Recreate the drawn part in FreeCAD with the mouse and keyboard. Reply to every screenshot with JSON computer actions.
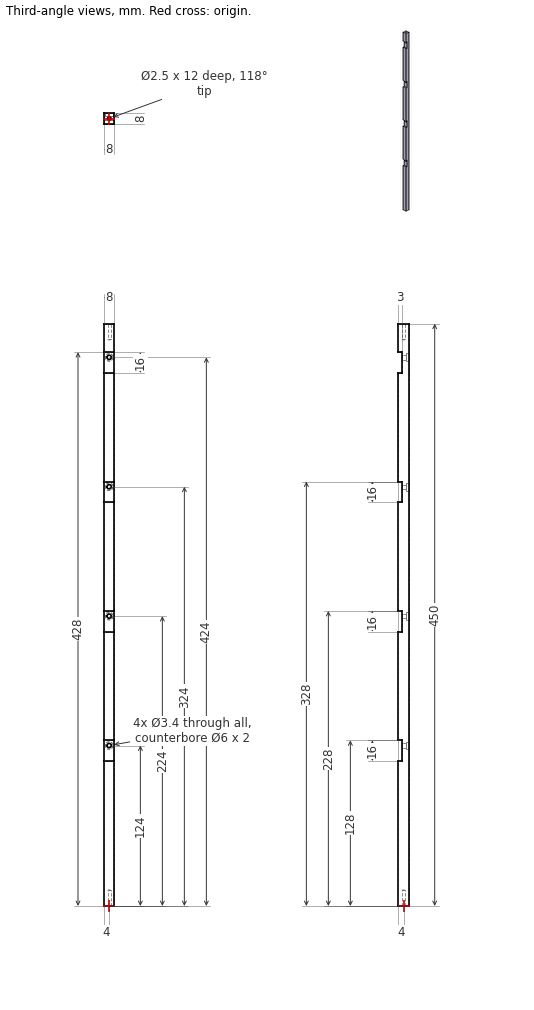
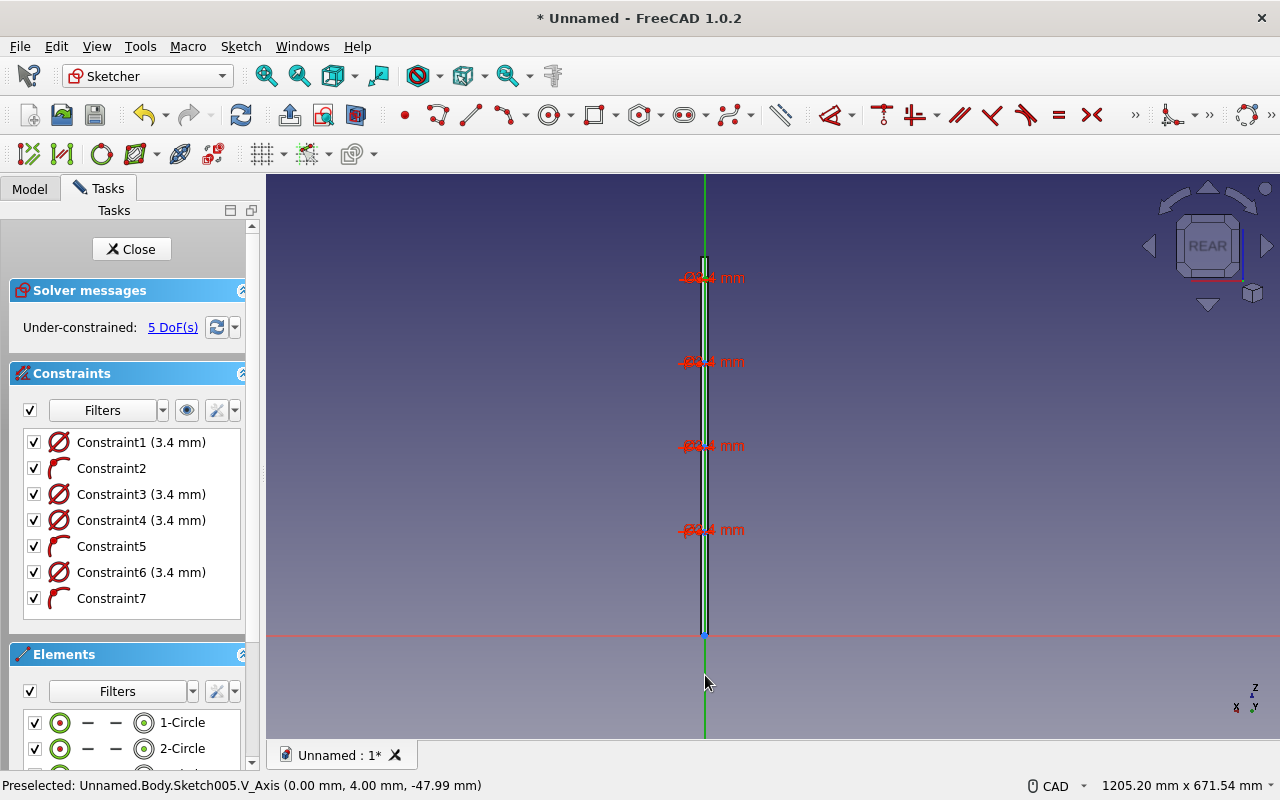
{"action": "key", "text": "c"}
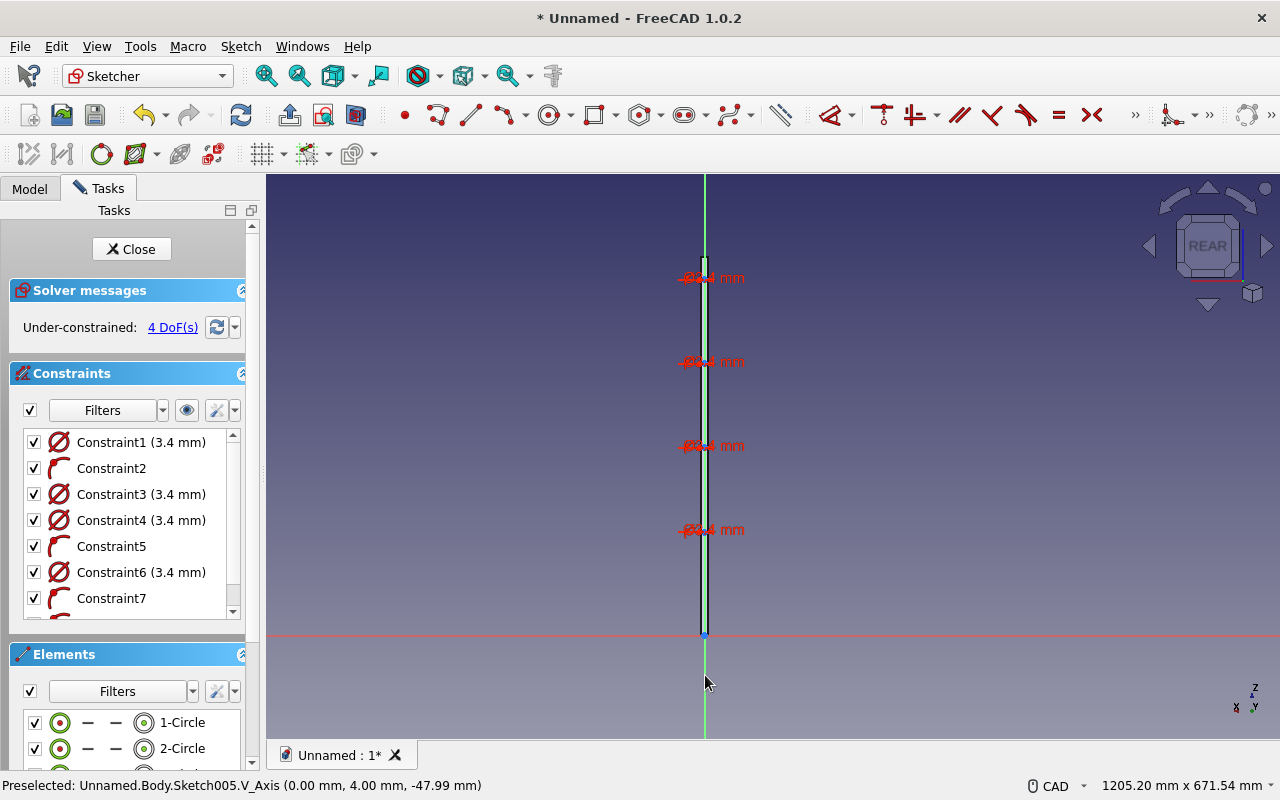
{"action": "key", "text": "d"}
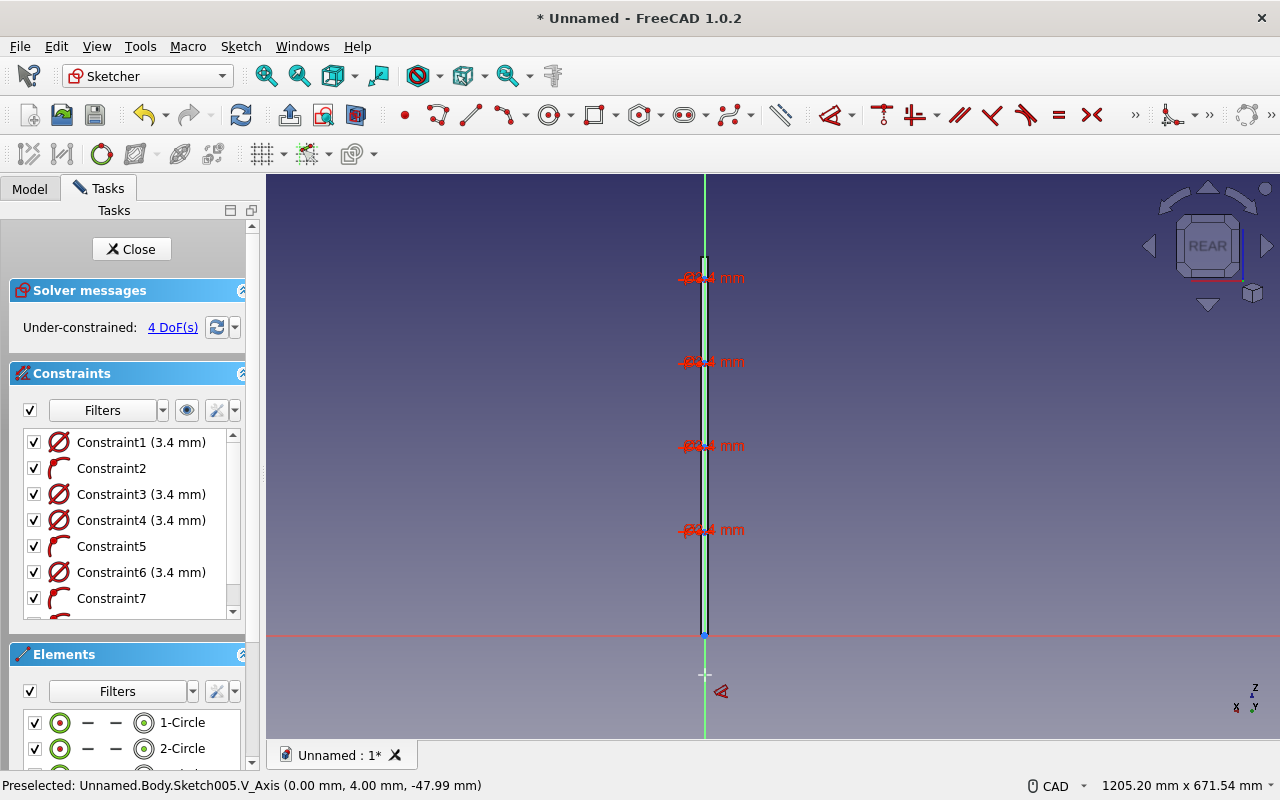
{"action": "left_click", "coordinate": [705, 532]}
{"action": "left_click", "coordinate": [739, 584]}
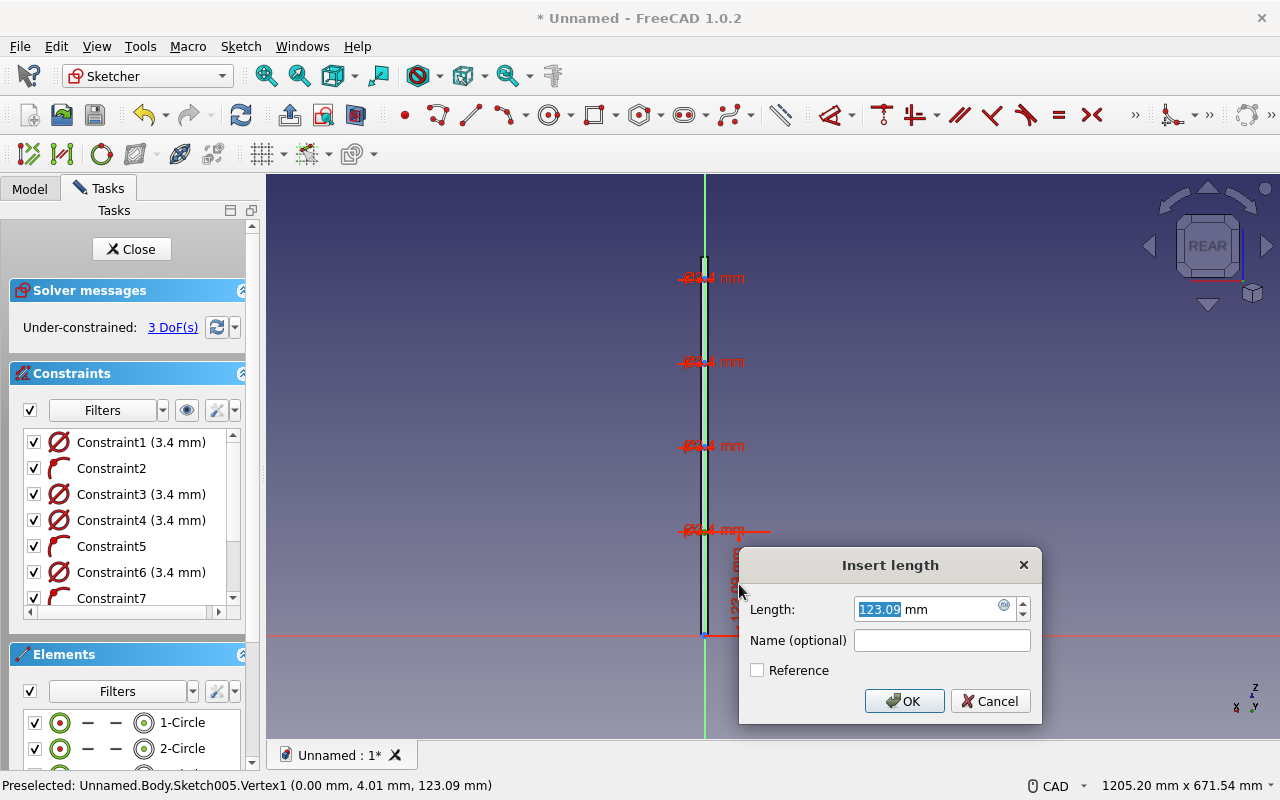
{"action": "type", "text": "124"}
{"action": "key", "text": "Return"}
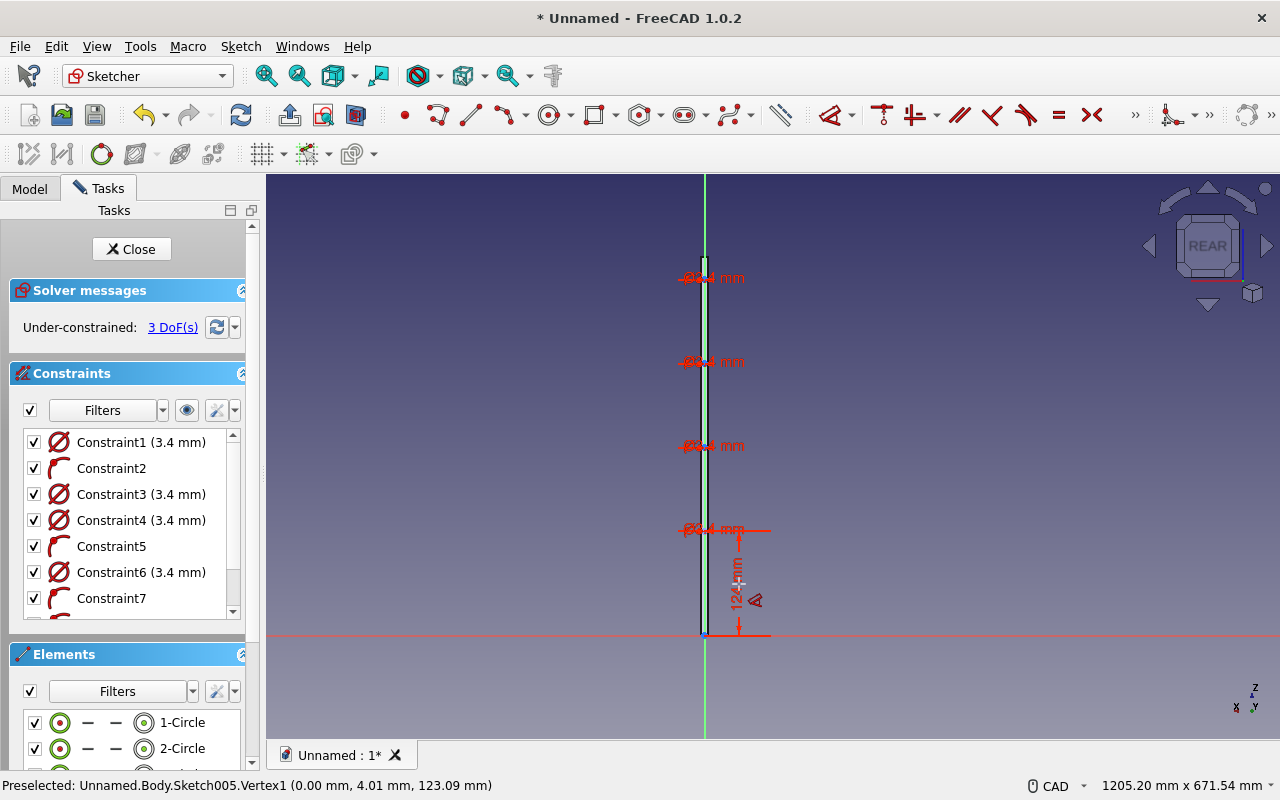
{"action": "left_click", "coordinate": [705, 448]}
{"action": "left_click", "coordinate": [739, 542]}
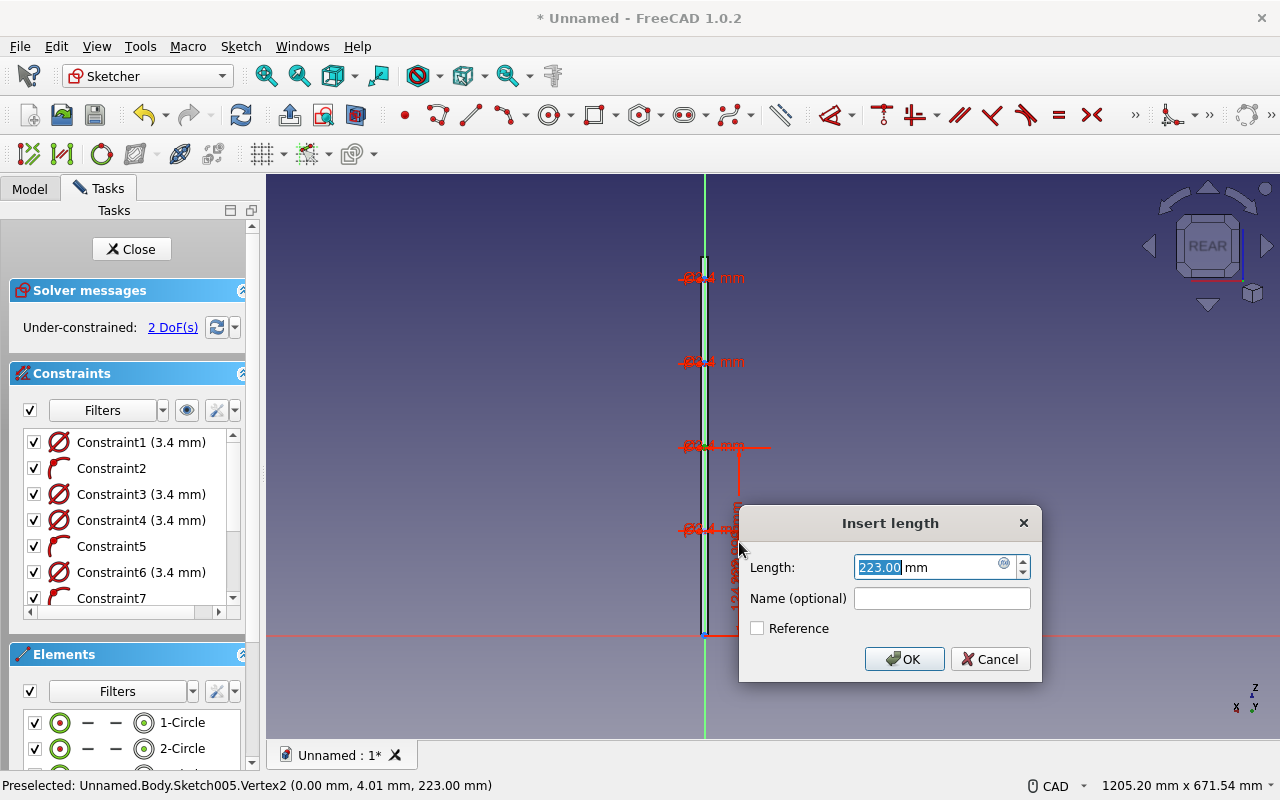
{"action": "type", "text": "224"}
{"action": "key", "text": "Return"}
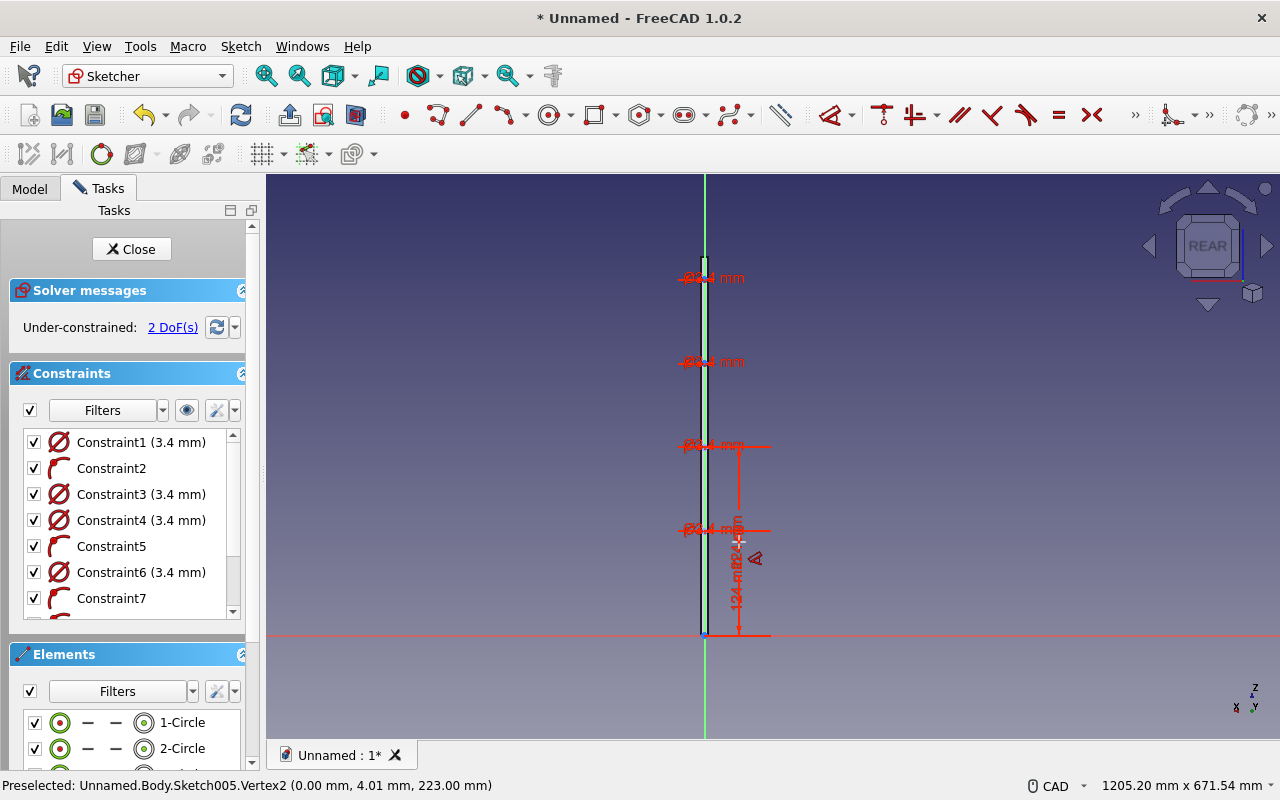
{"action": "left_click", "coordinate": [705, 364]}
{"action": "left_click", "coordinate": [739, 500]}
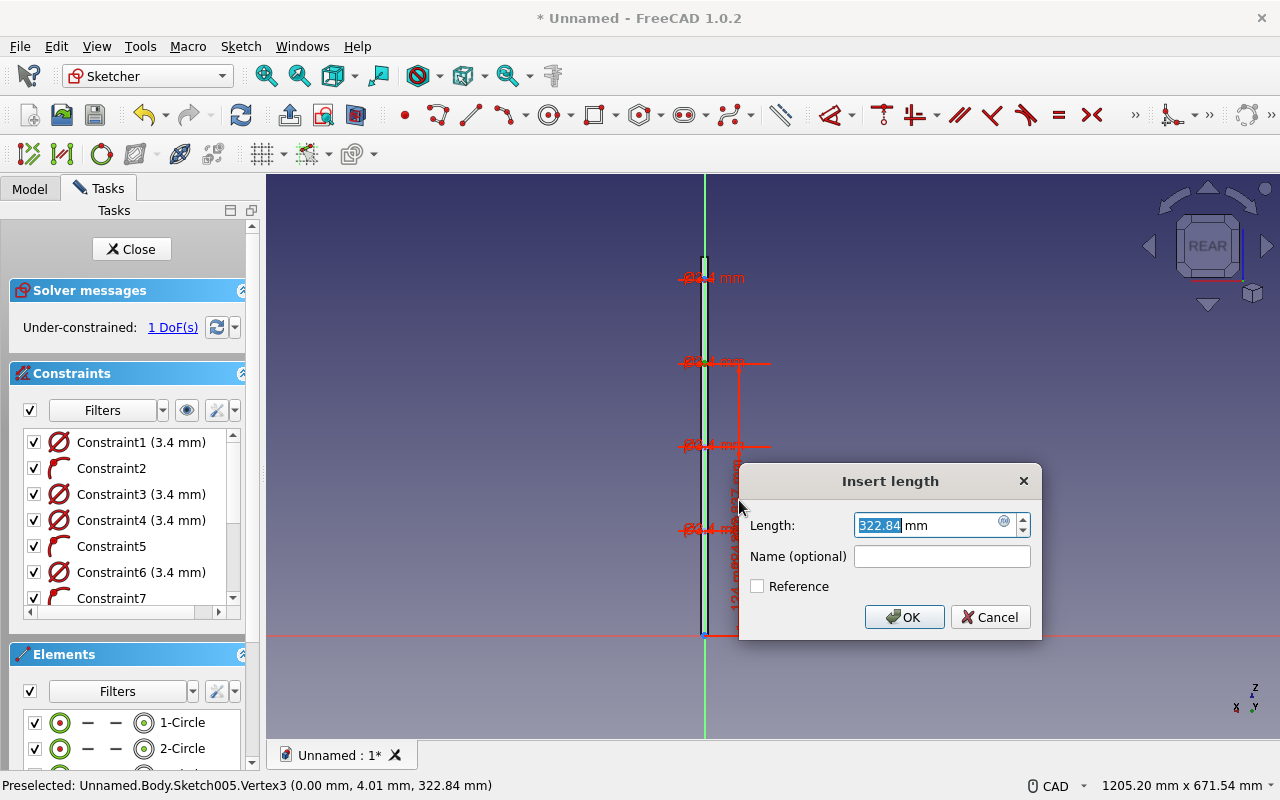
{"action": "type", "text": "324"}
{"action": "key", "text": "Return"}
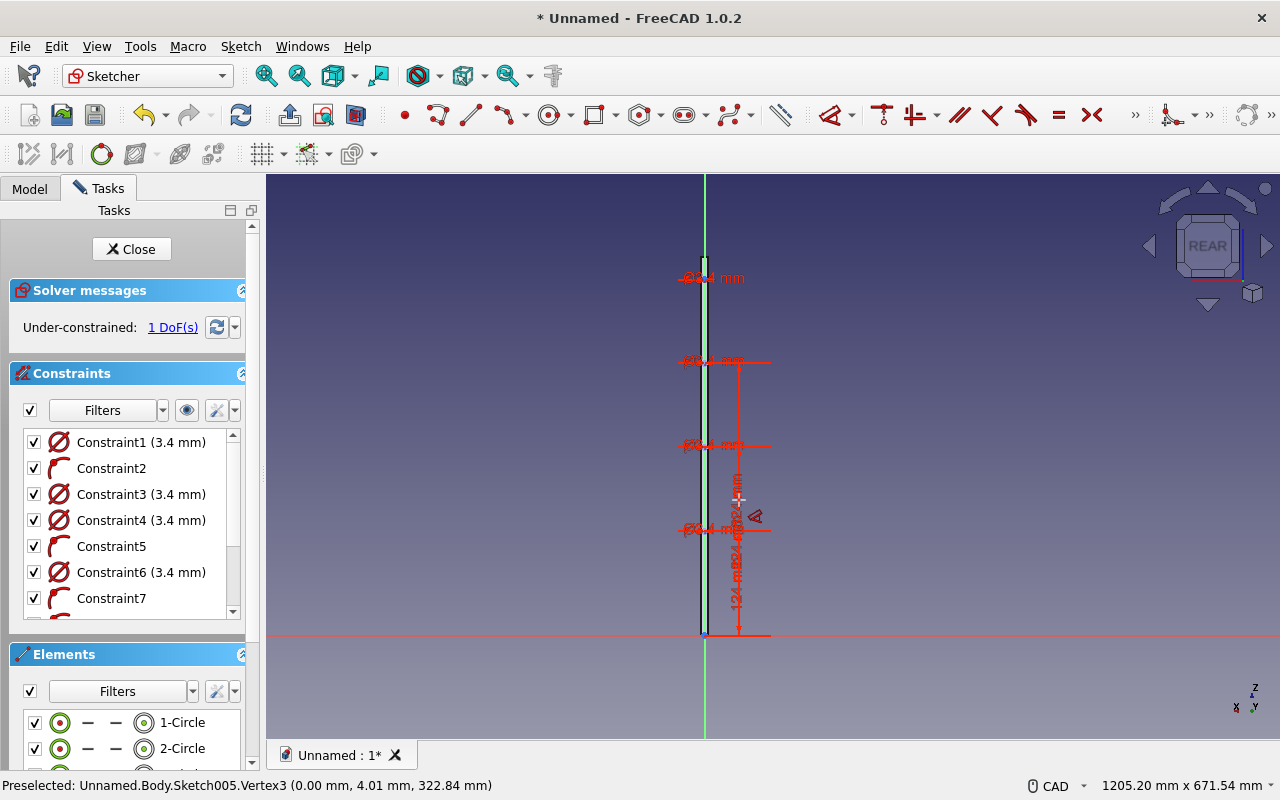
{"action": "left_click", "coordinate": [705, 280]}
{"action": "left_click", "coordinate": [739, 458]}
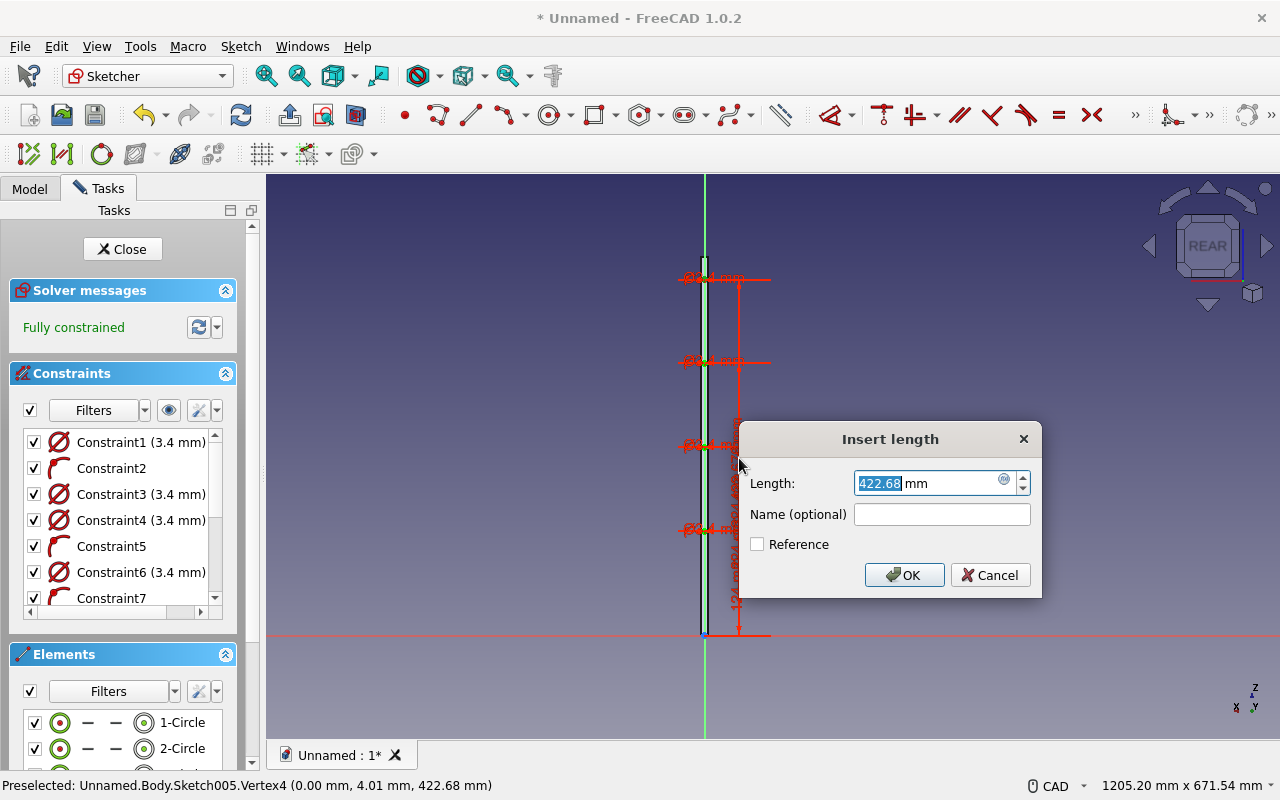
{"action": "type", "text": "424"}
{"action": "key", "text": "Return"}
{"action": "key", "text": "Escape"}